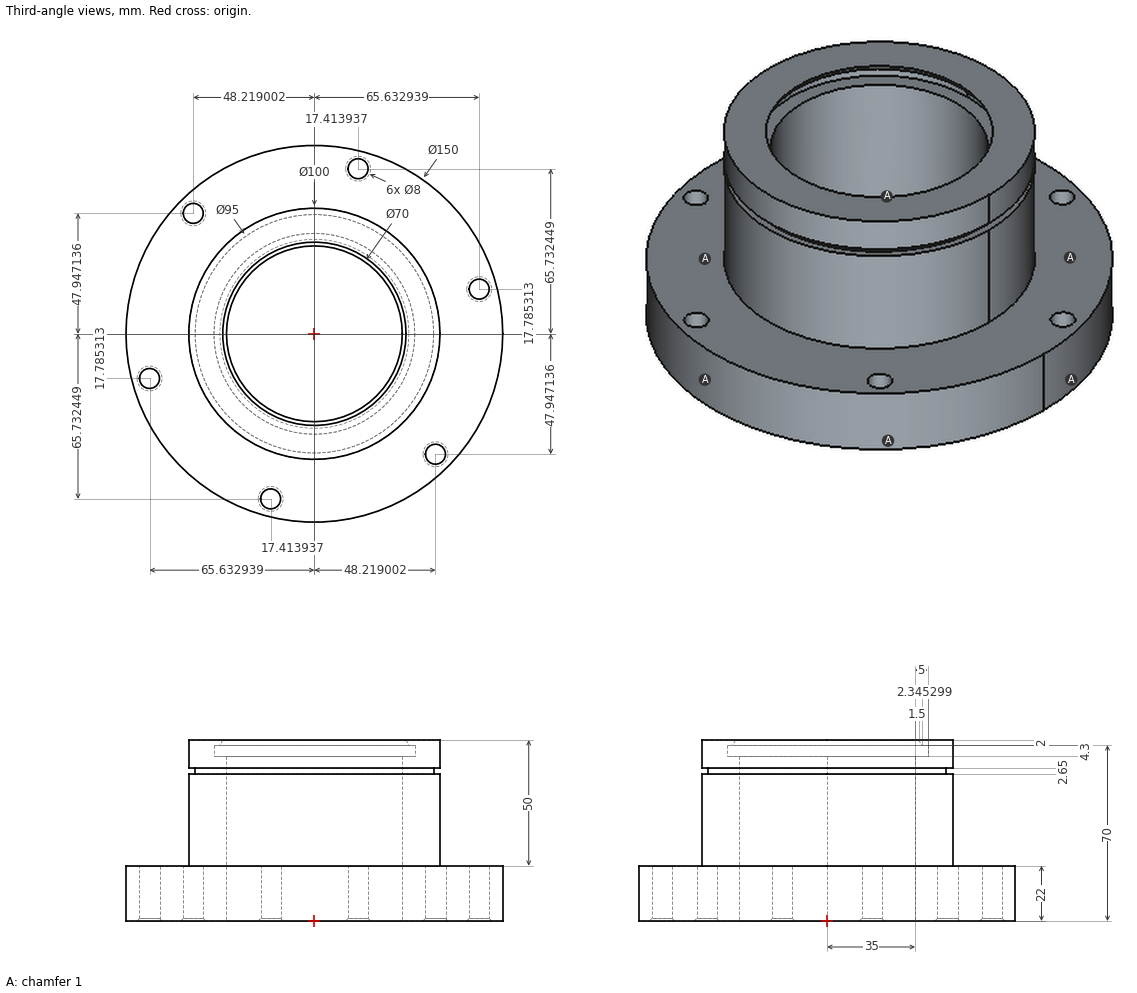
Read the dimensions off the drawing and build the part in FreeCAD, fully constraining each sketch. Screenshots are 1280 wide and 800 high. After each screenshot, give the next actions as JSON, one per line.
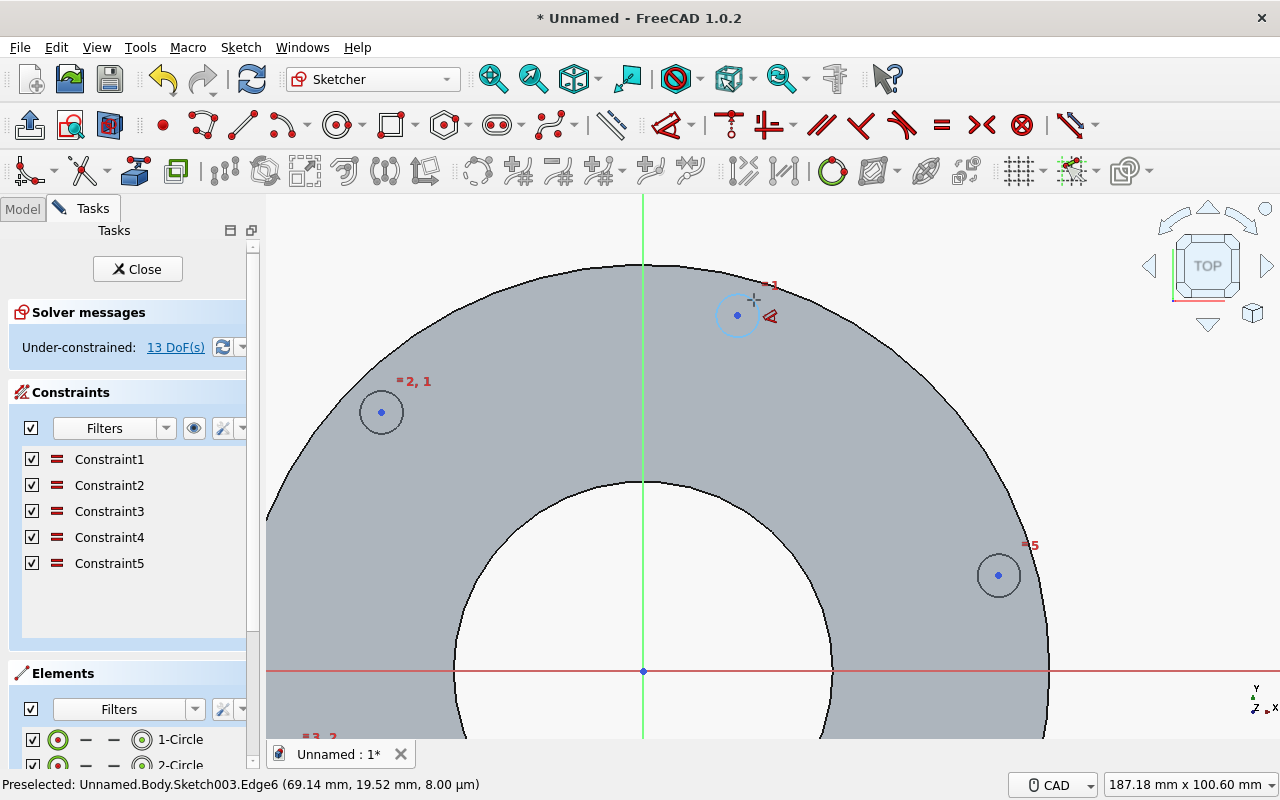
{"action": "left_click", "coordinate": [753, 301]}
{"action": "left_click", "coordinate": [776, 279]}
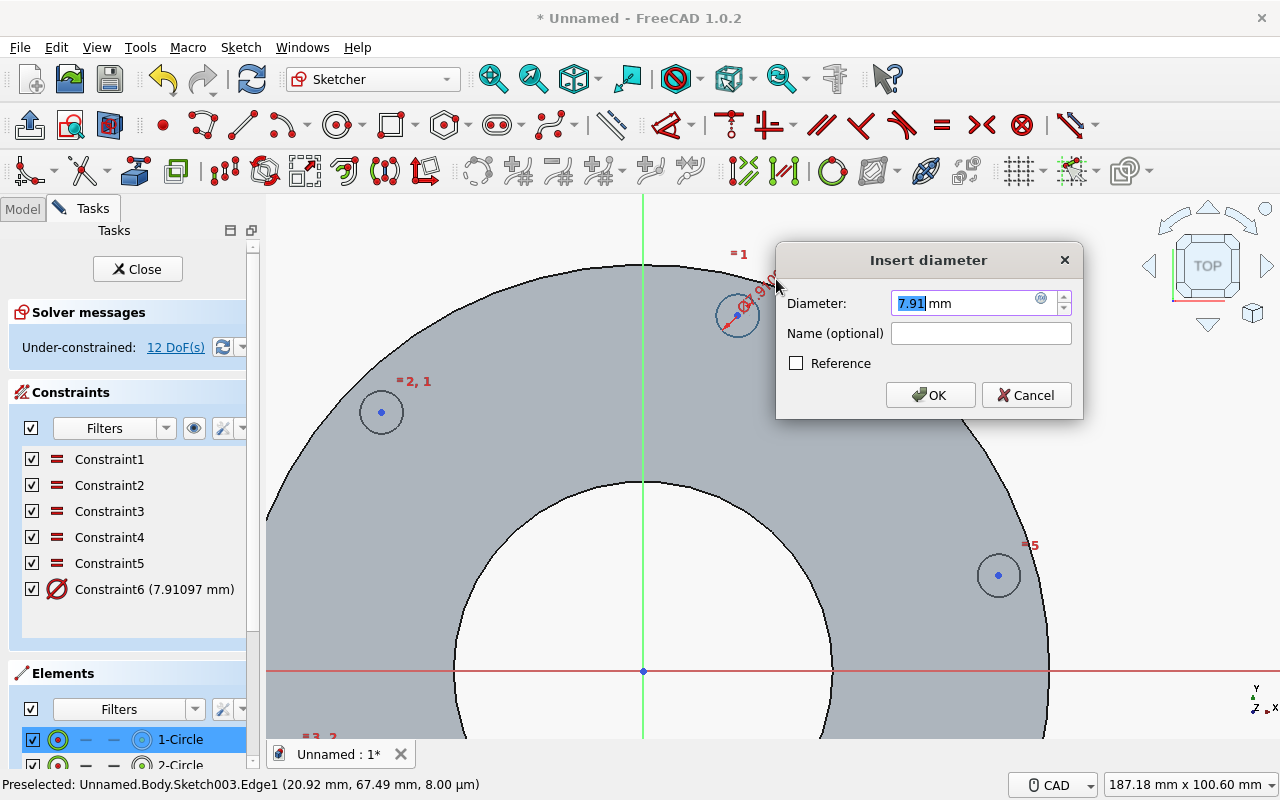
{"action": "type", "text": "8"}
{"action": "key", "text": "Return"}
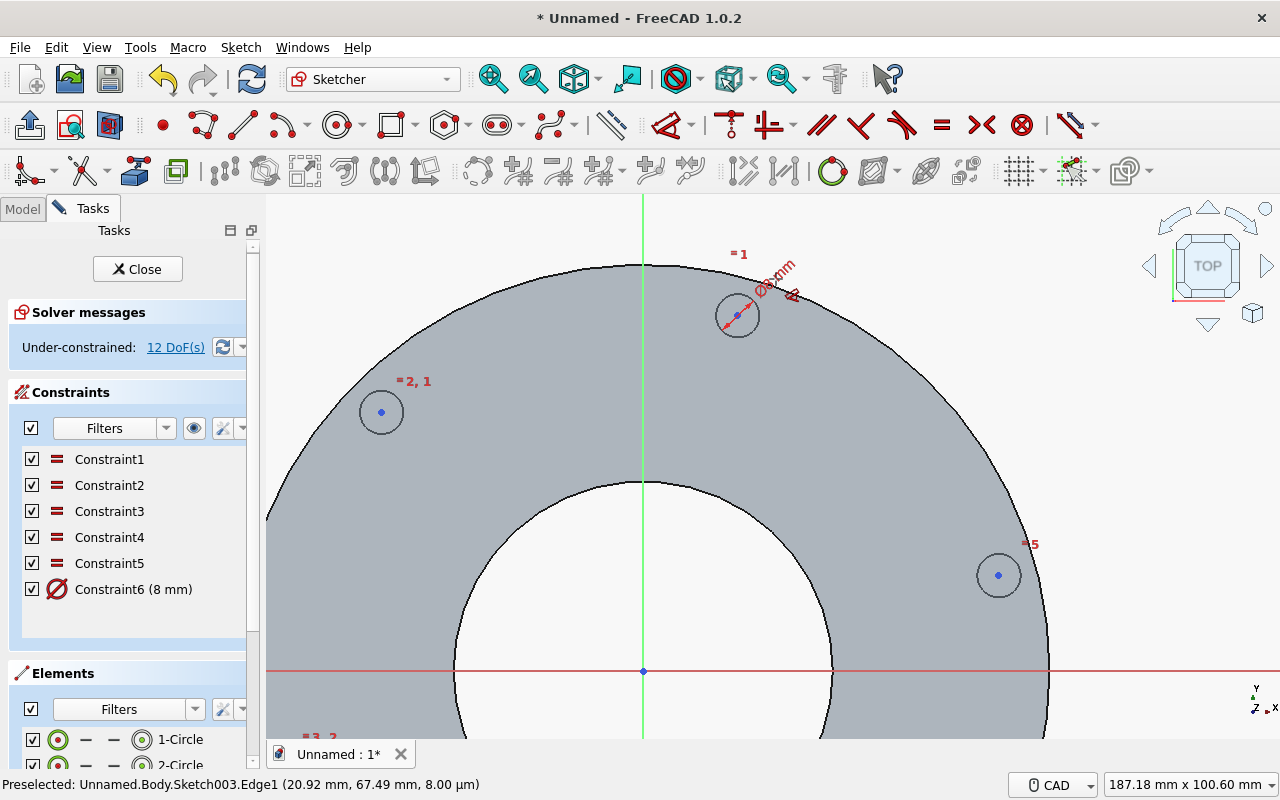
{"action": "left_click", "coordinate": [738, 316]}
{"action": "left_click", "coordinate": [691, 282]}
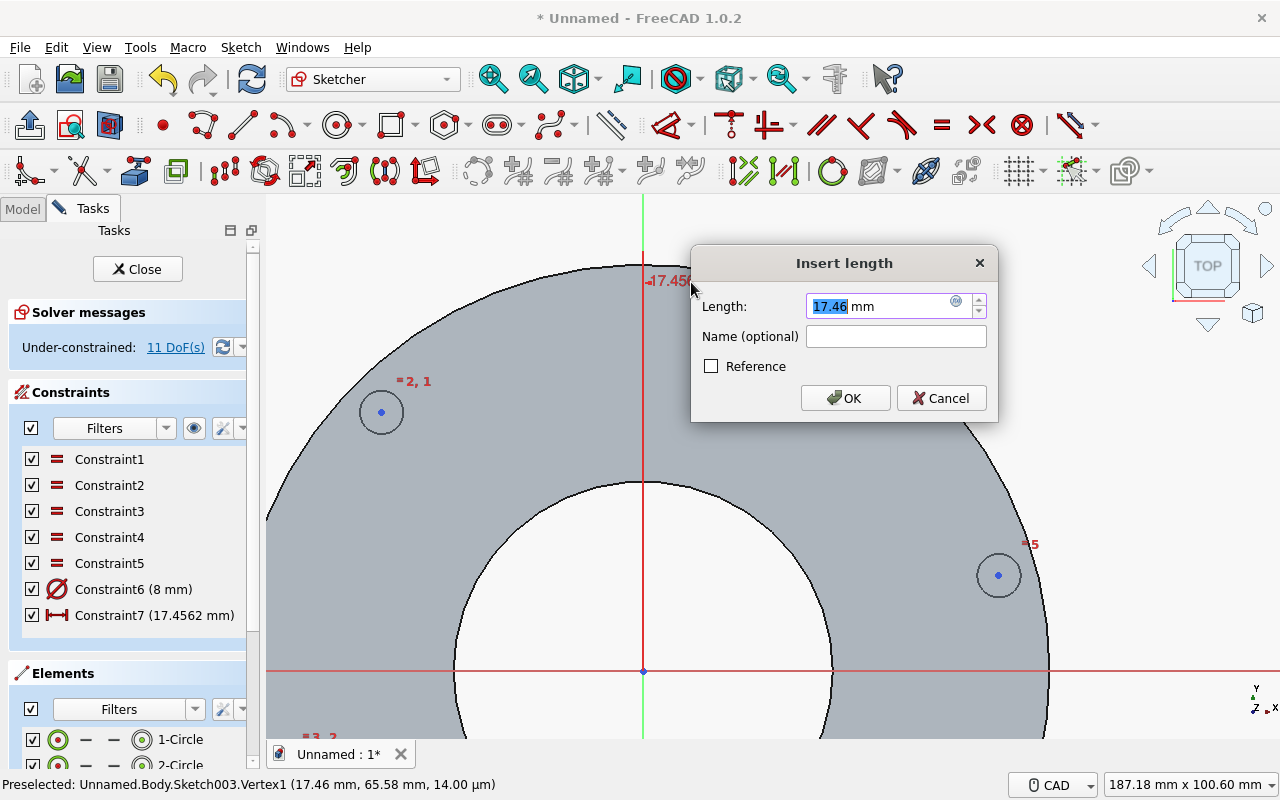
{"action": "type", "text": "17.413937"}
{"action": "key", "text": "Return"}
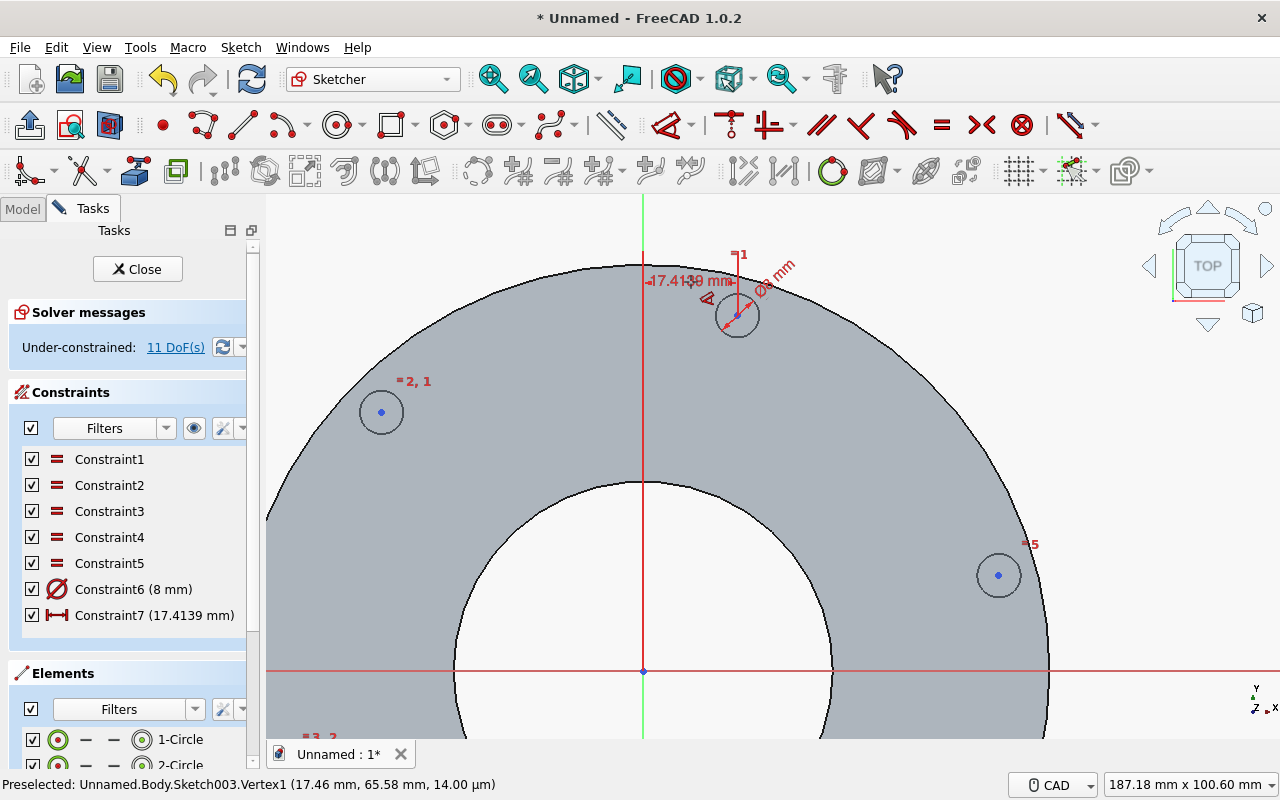
{"action": "left_click", "coordinate": [738, 316]}
{"action": "left_click", "coordinate": [772, 493]}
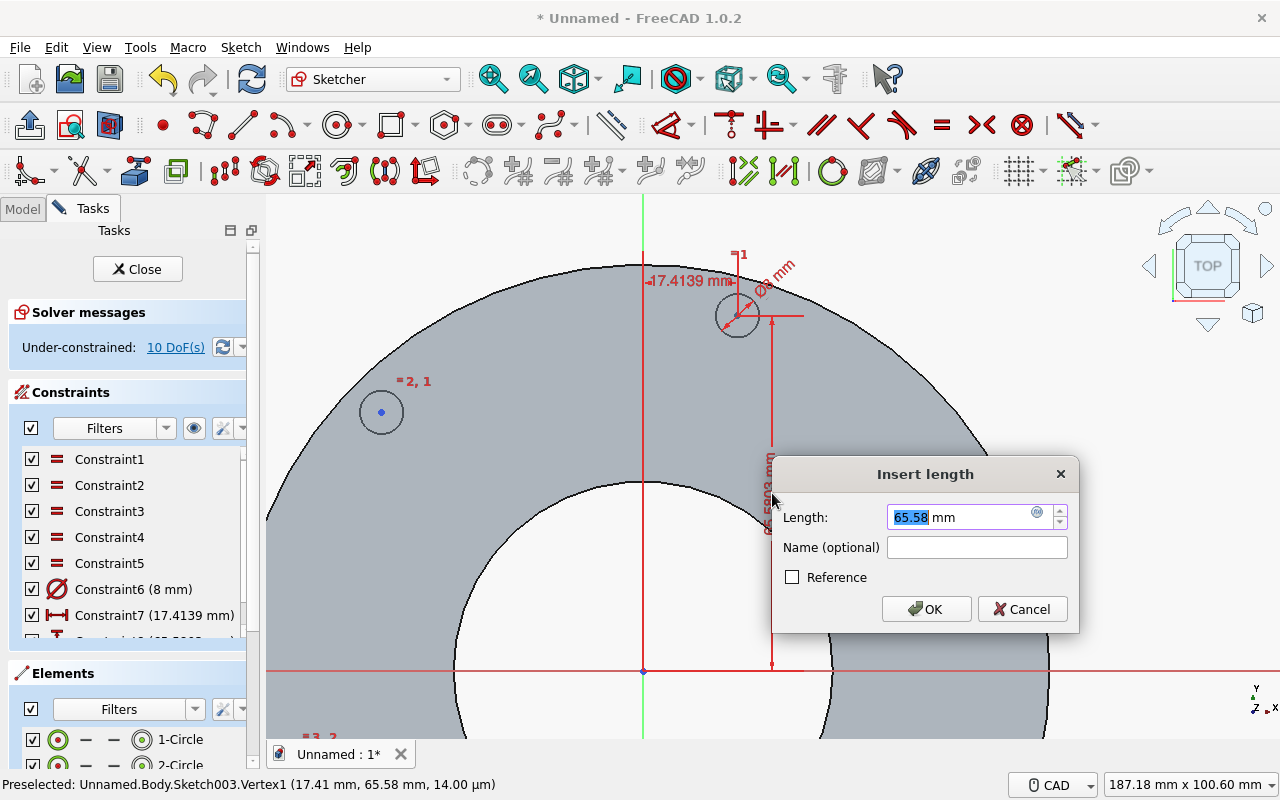
{"action": "type", "text": "65.732449"}
{"action": "key", "text": "Return"}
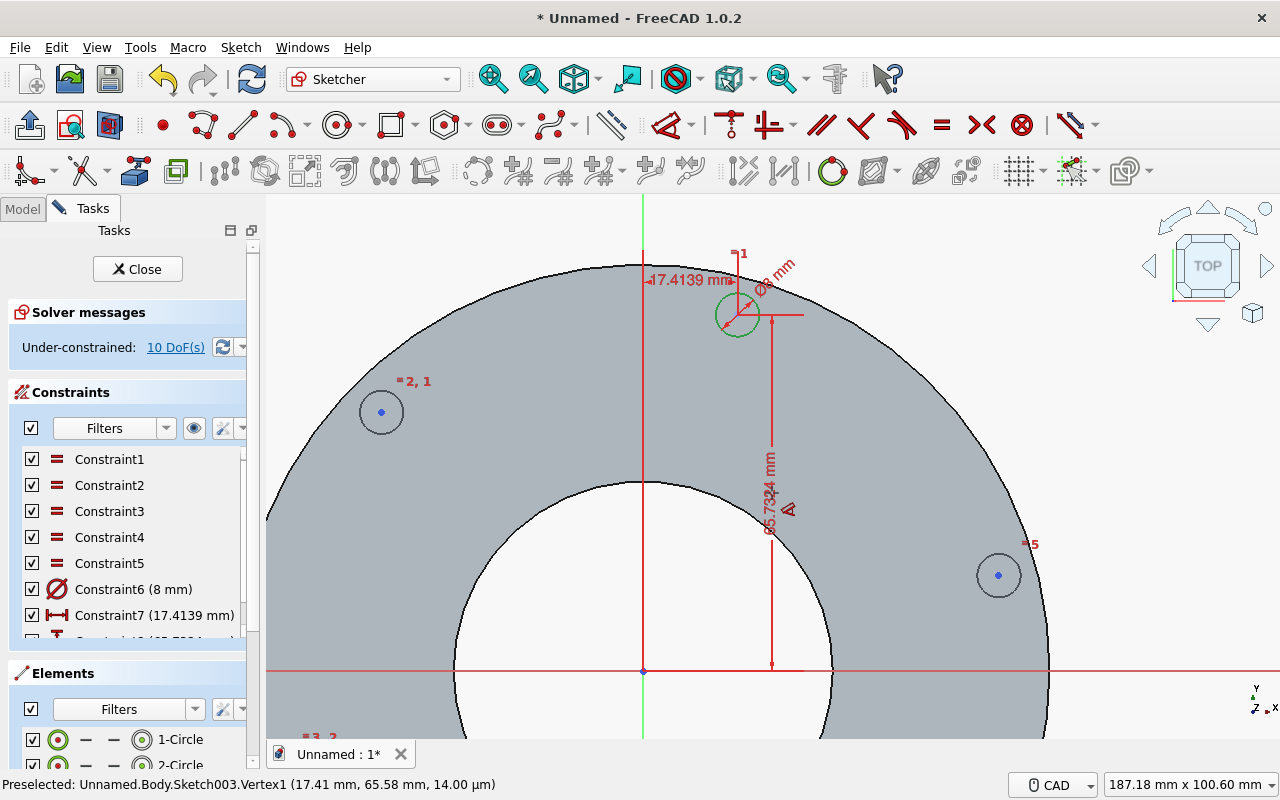
{"action": "left_click", "coordinate": [382, 412]}
{"action": "left_click", "coordinate": [512, 378]}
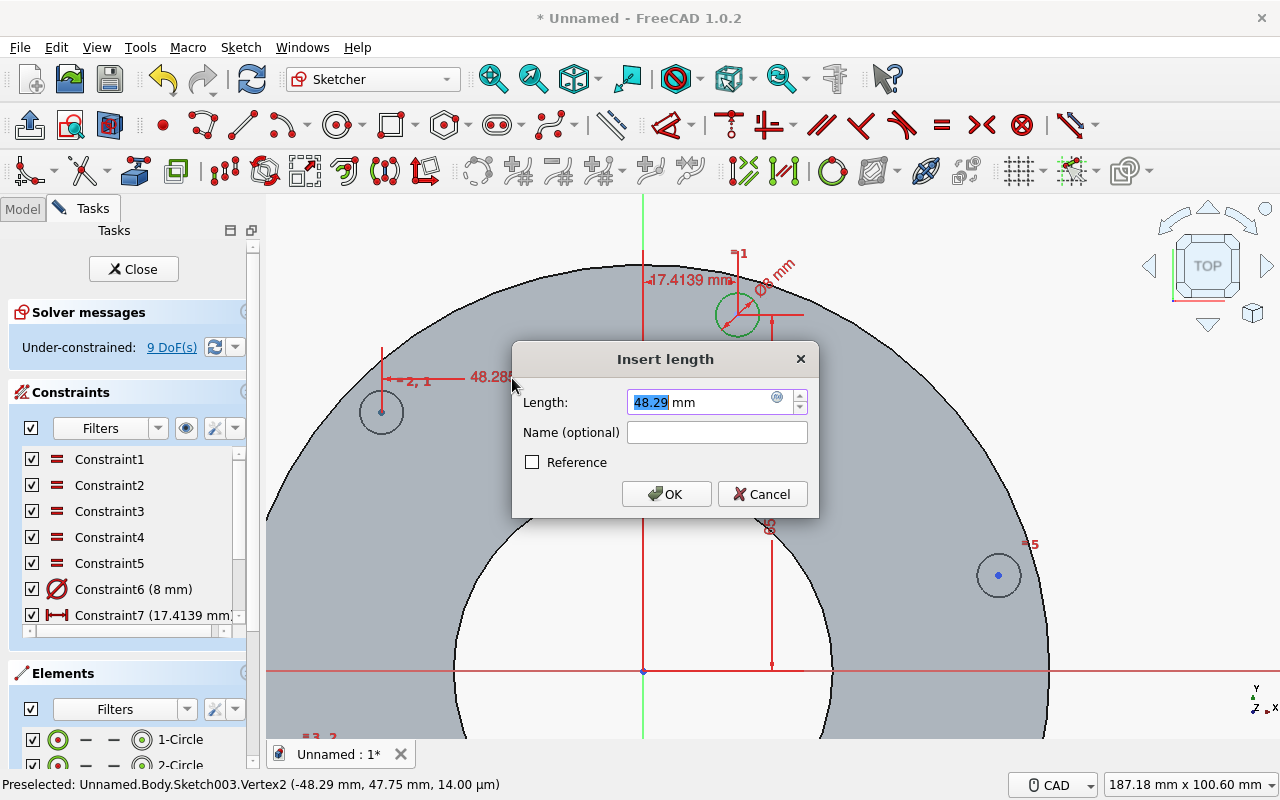
{"action": "type", "text": "48.219002"}
{"action": "key", "text": "Return"}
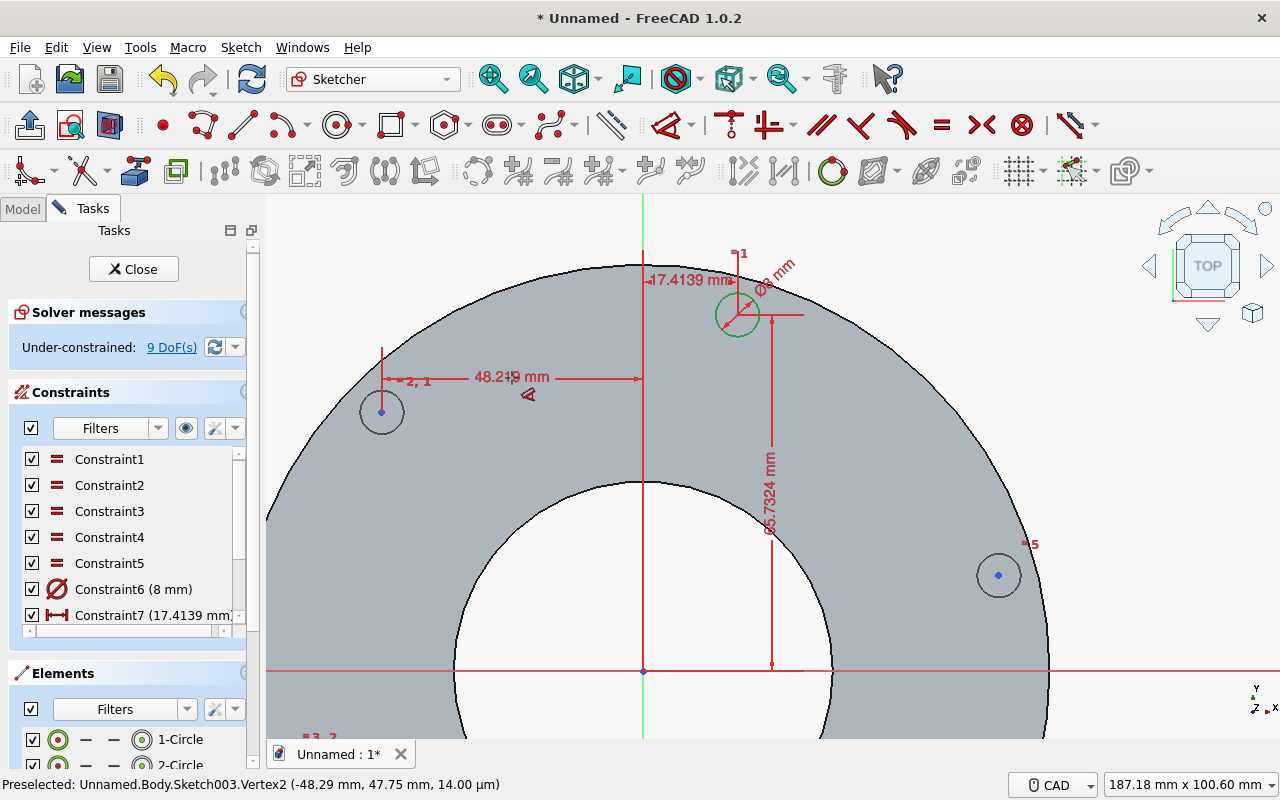
{"action": "left_click", "coordinate": [382, 412]}
{"action": "left_click", "coordinate": [348, 542]}